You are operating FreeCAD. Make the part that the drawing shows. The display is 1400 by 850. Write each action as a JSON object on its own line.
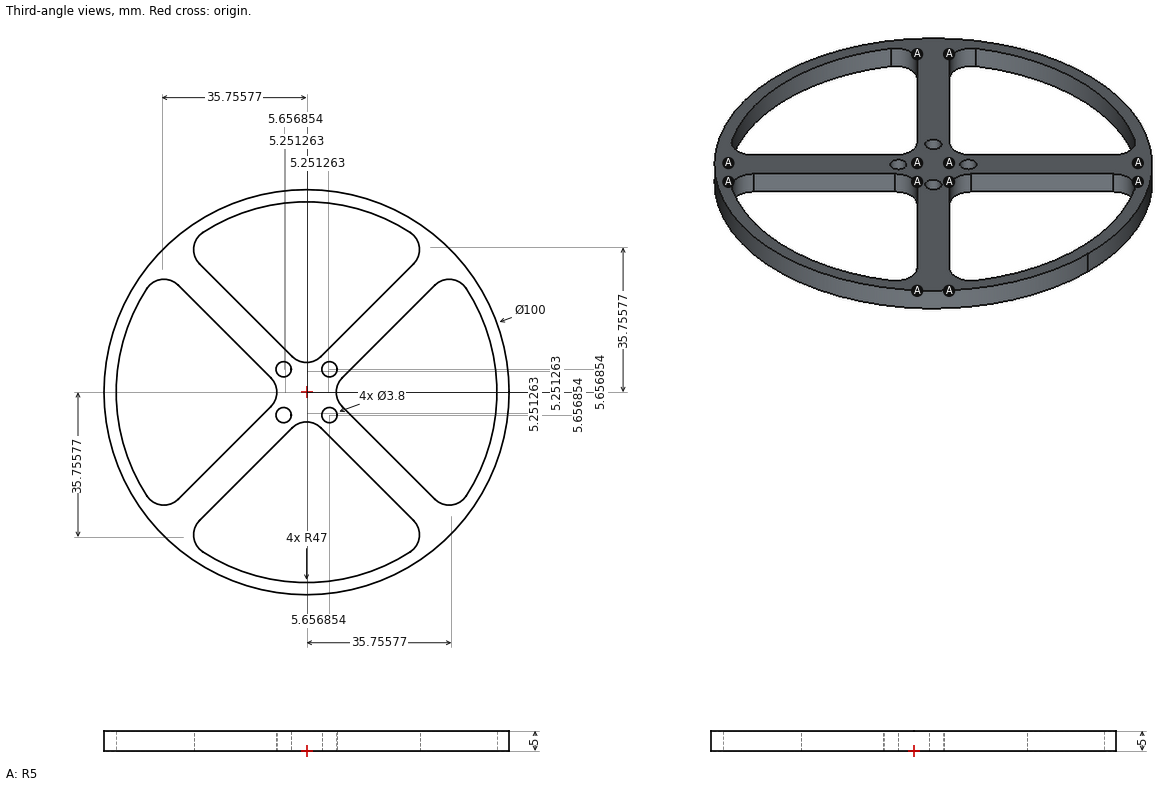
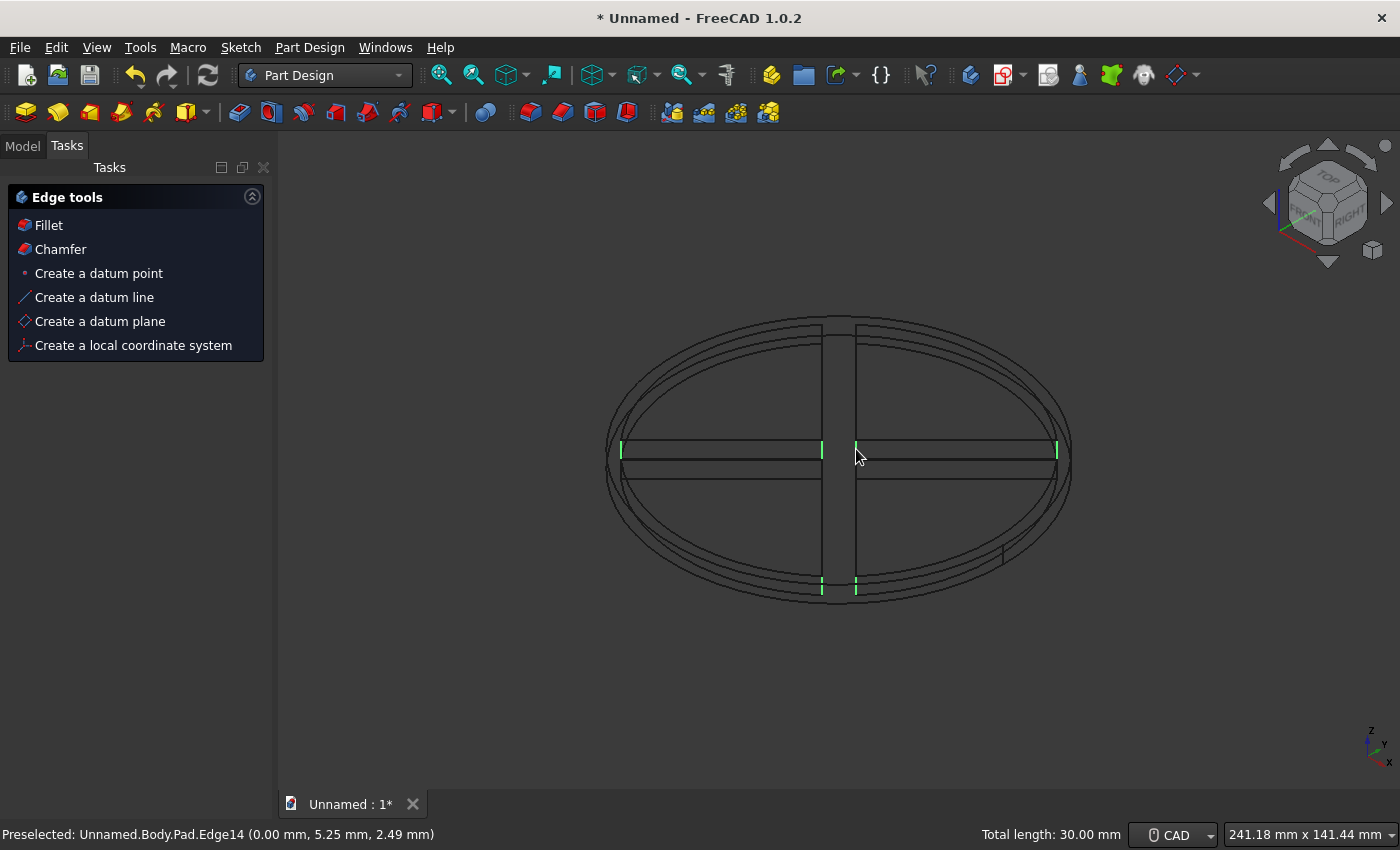
{"action": "key", "text": "2"}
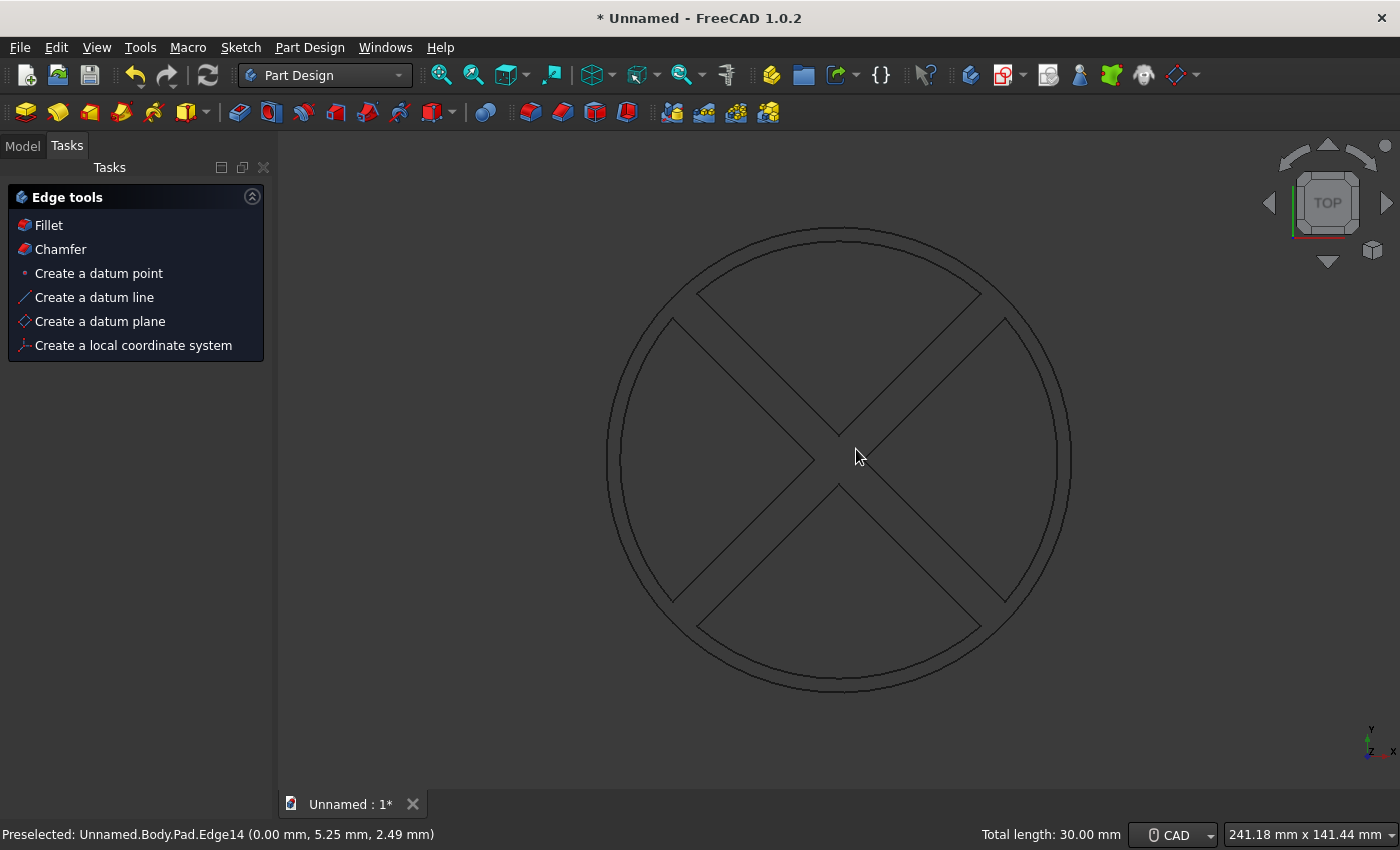
{"action": "key", "text": "1"}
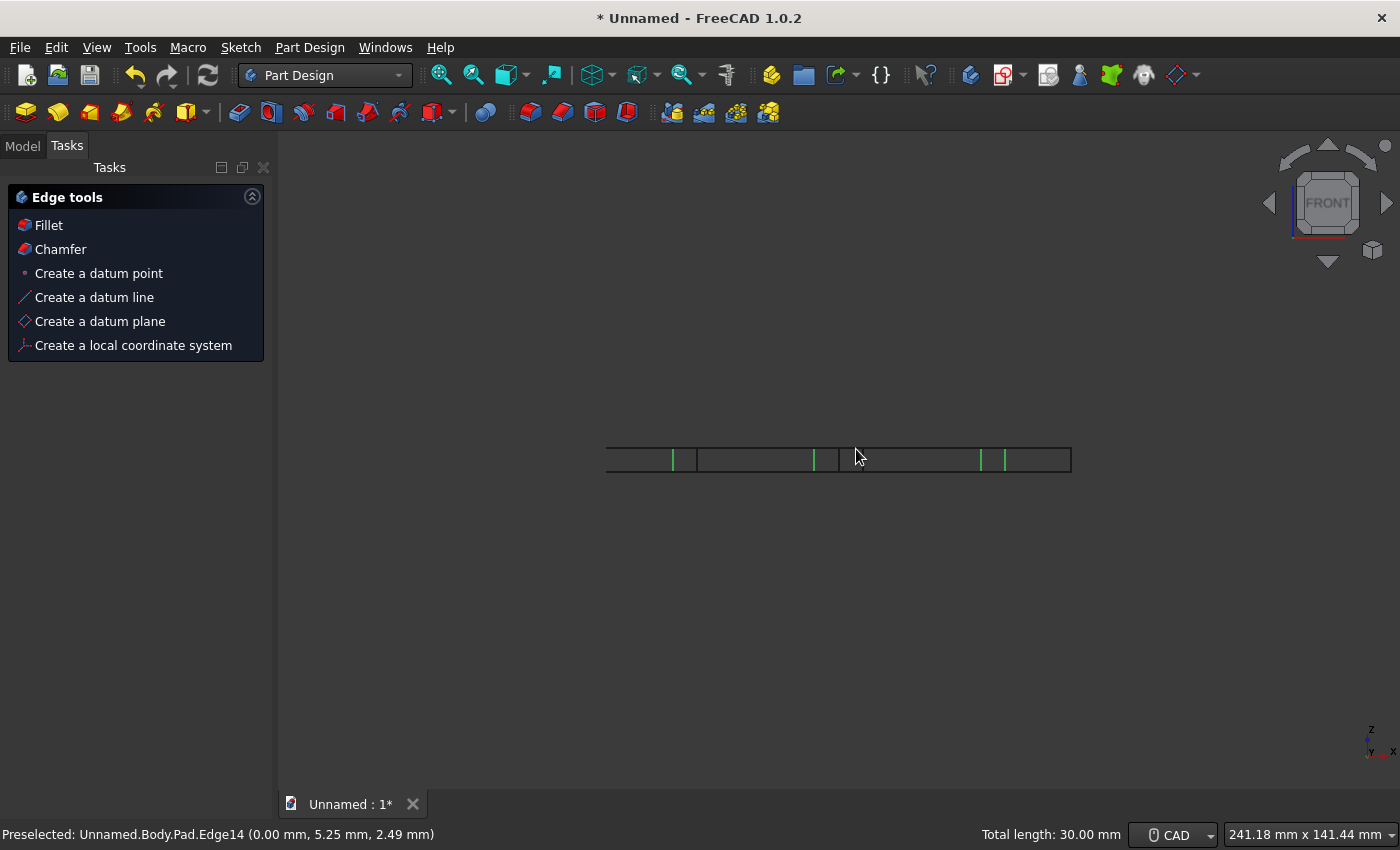
{"action": "left_click", "coordinate": [442, 76]}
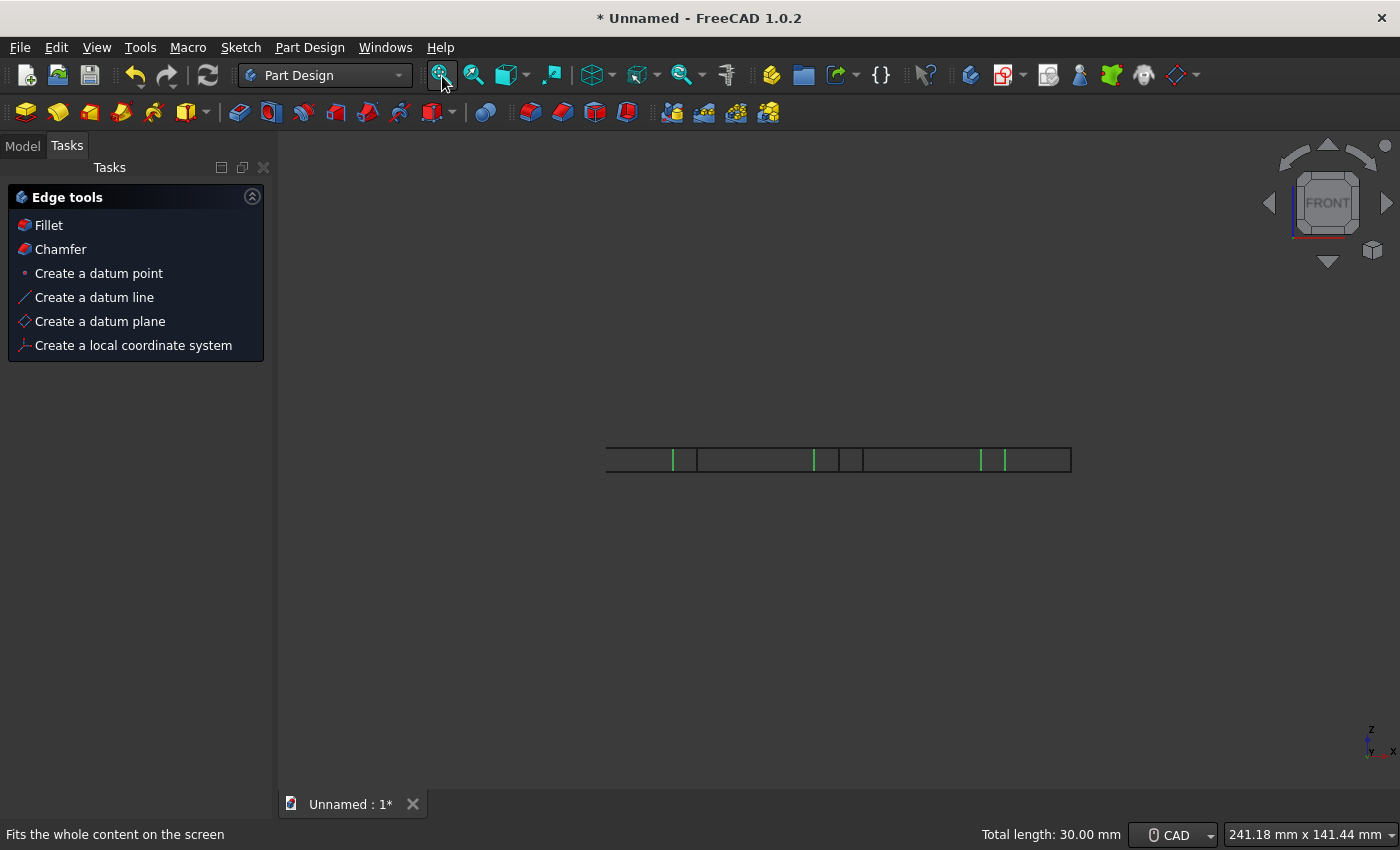
{"action": "left_click", "coordinate": [863, 459], "text": "ctrl"}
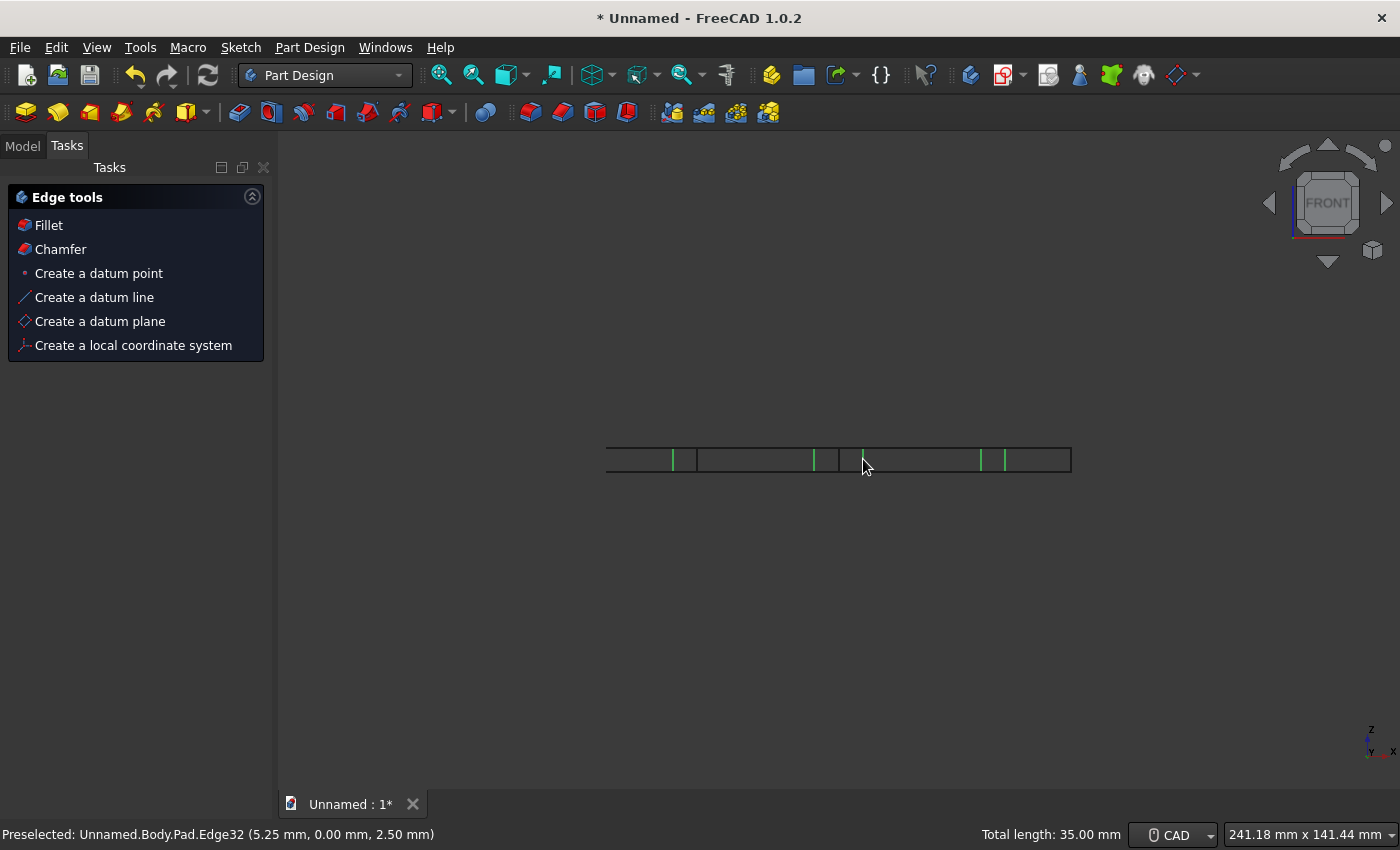
{"action": "left_click", "coordinate": [697, 459], "text": "ctrl"}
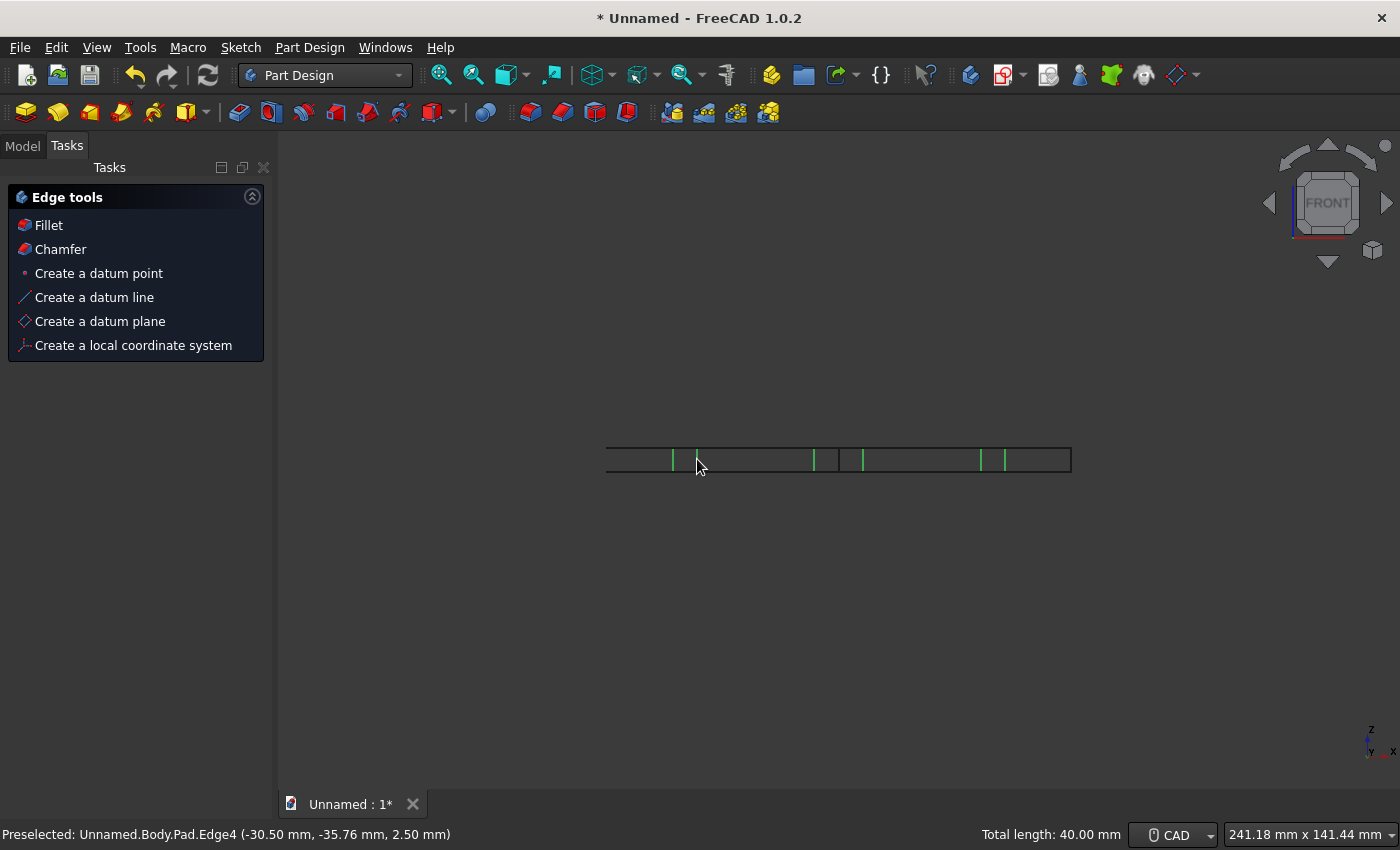
{"action": "left_click", "coordinate": [839, 459], "text": "ctrl"}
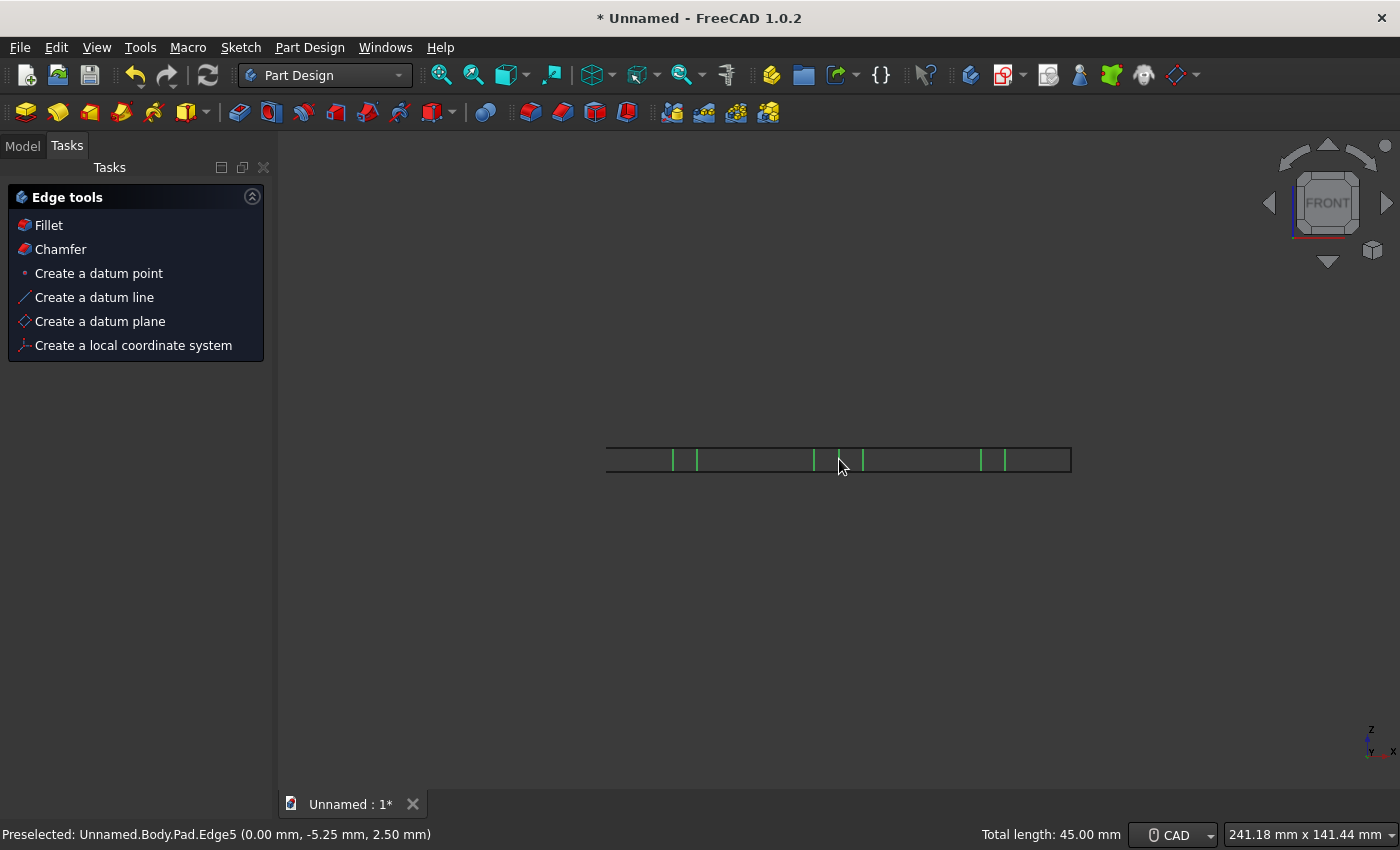
{"action": "key", "text": "3"}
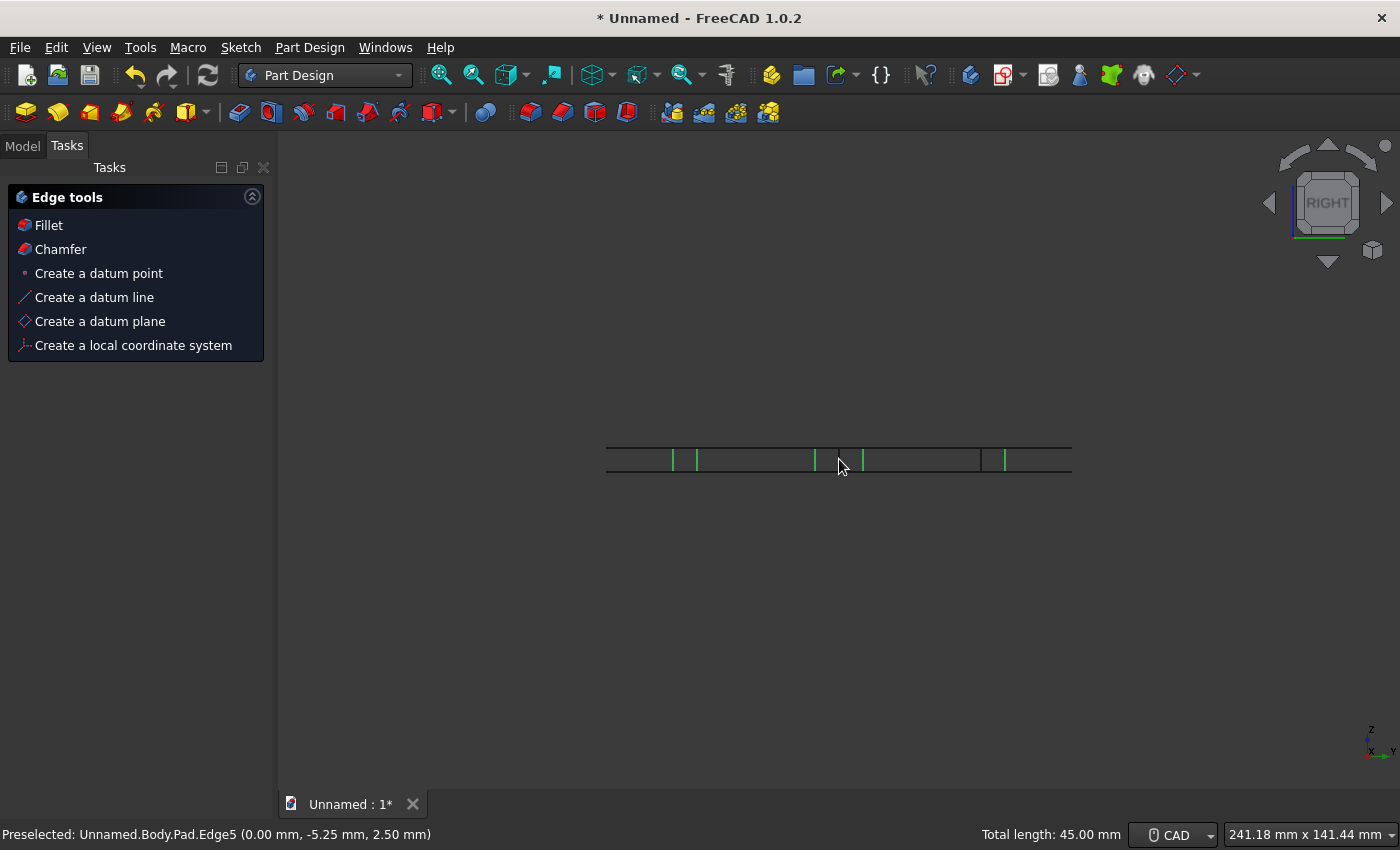
{"action": "left_click", "coordinate": [442, 76]}